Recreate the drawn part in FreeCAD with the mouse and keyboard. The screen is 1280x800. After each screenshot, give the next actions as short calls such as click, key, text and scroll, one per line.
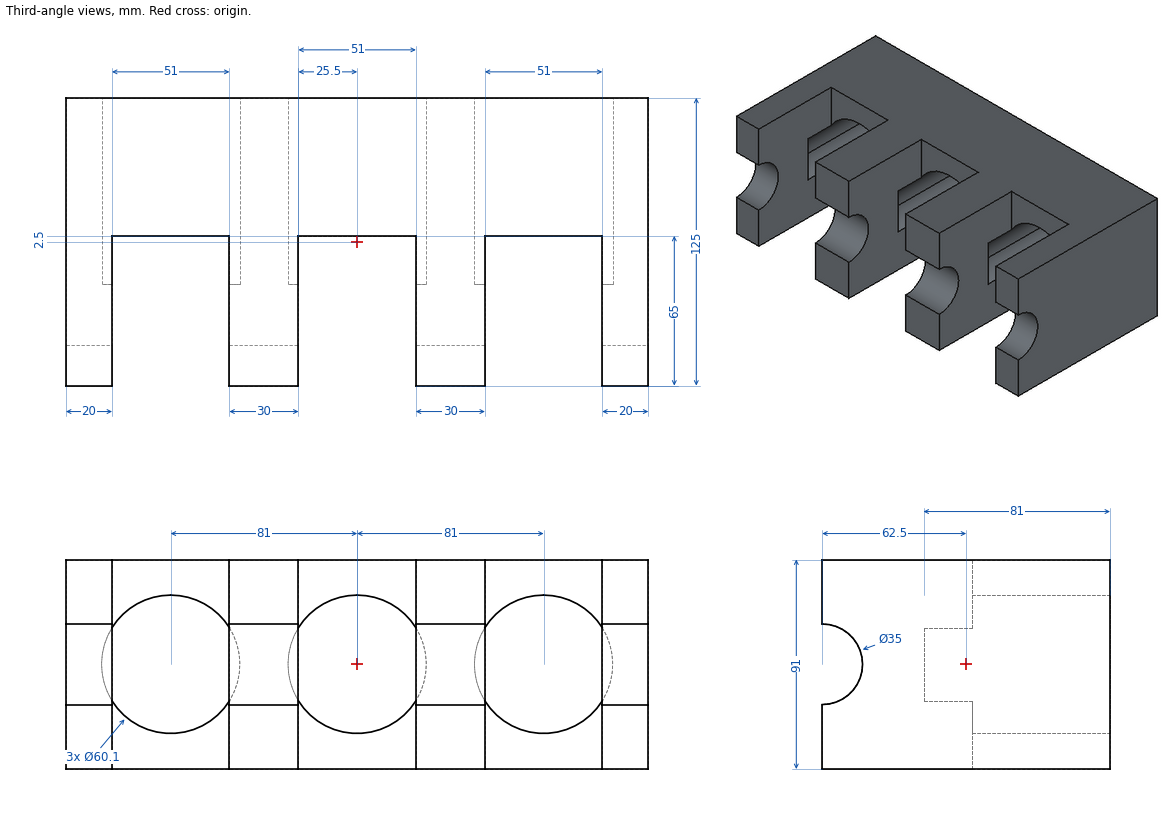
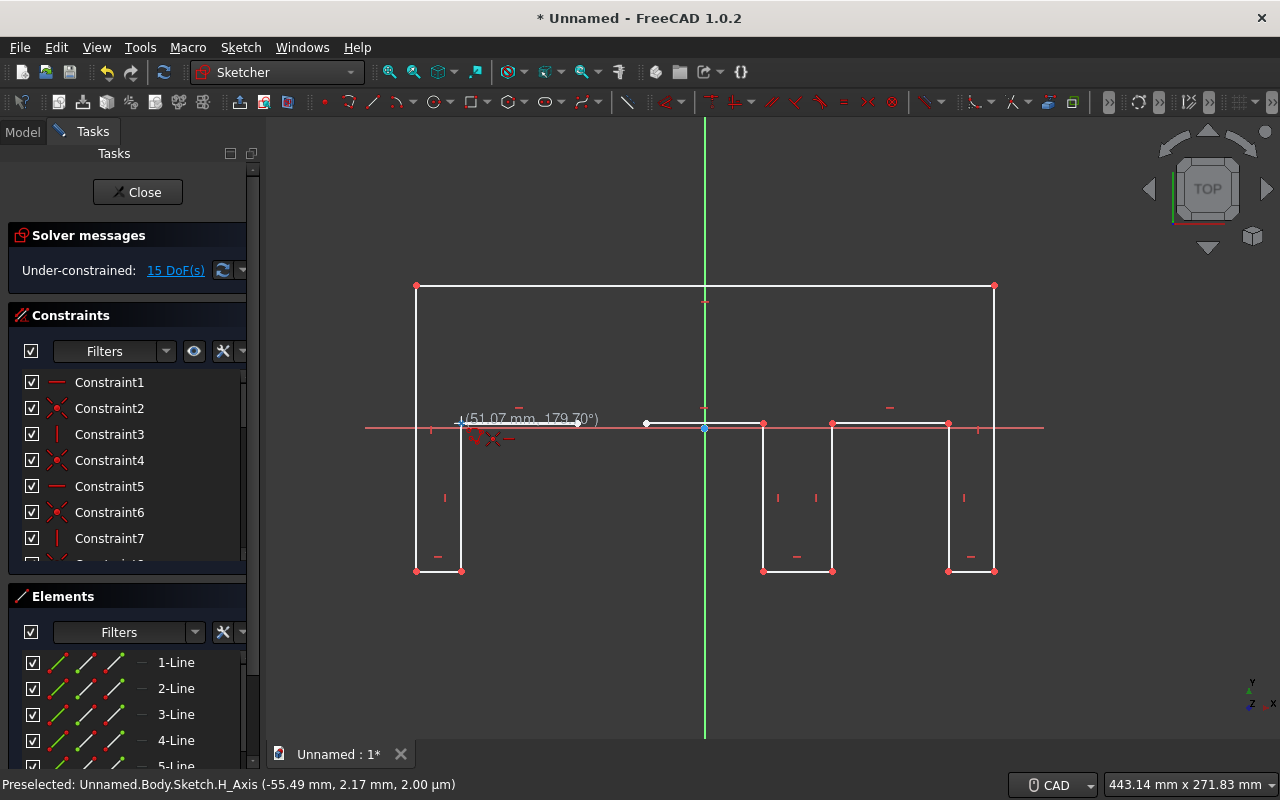
click(578, 571)
click(647, 571)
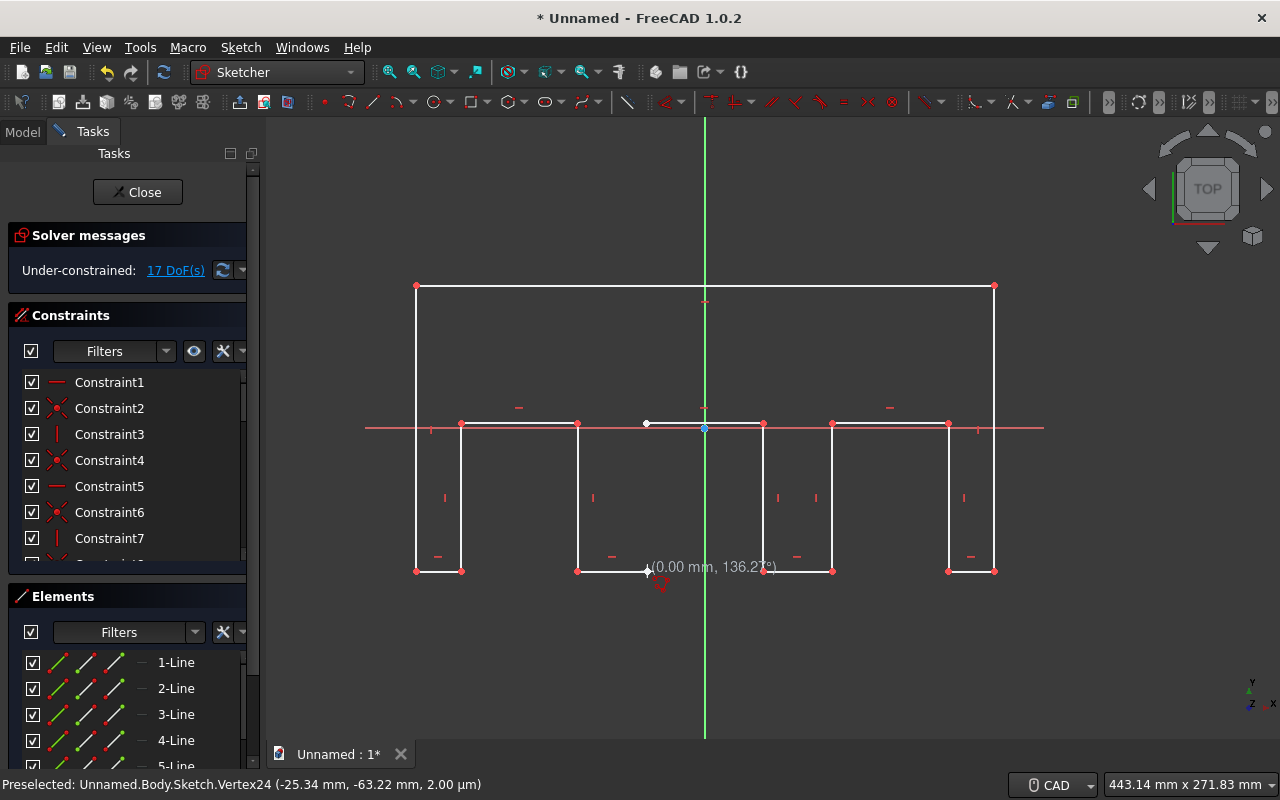
scroll(647, 423, up, 6)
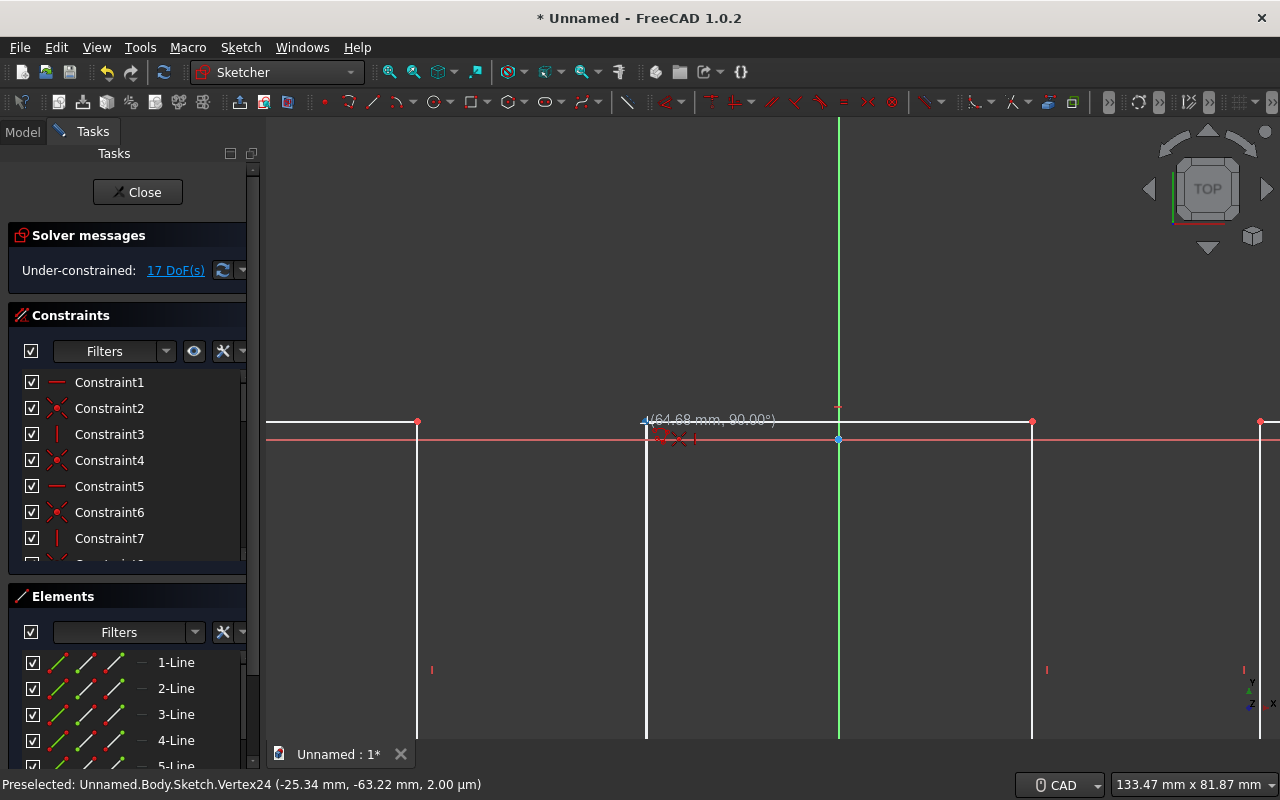
click(645, 422)
key(Escape)
key(Escape)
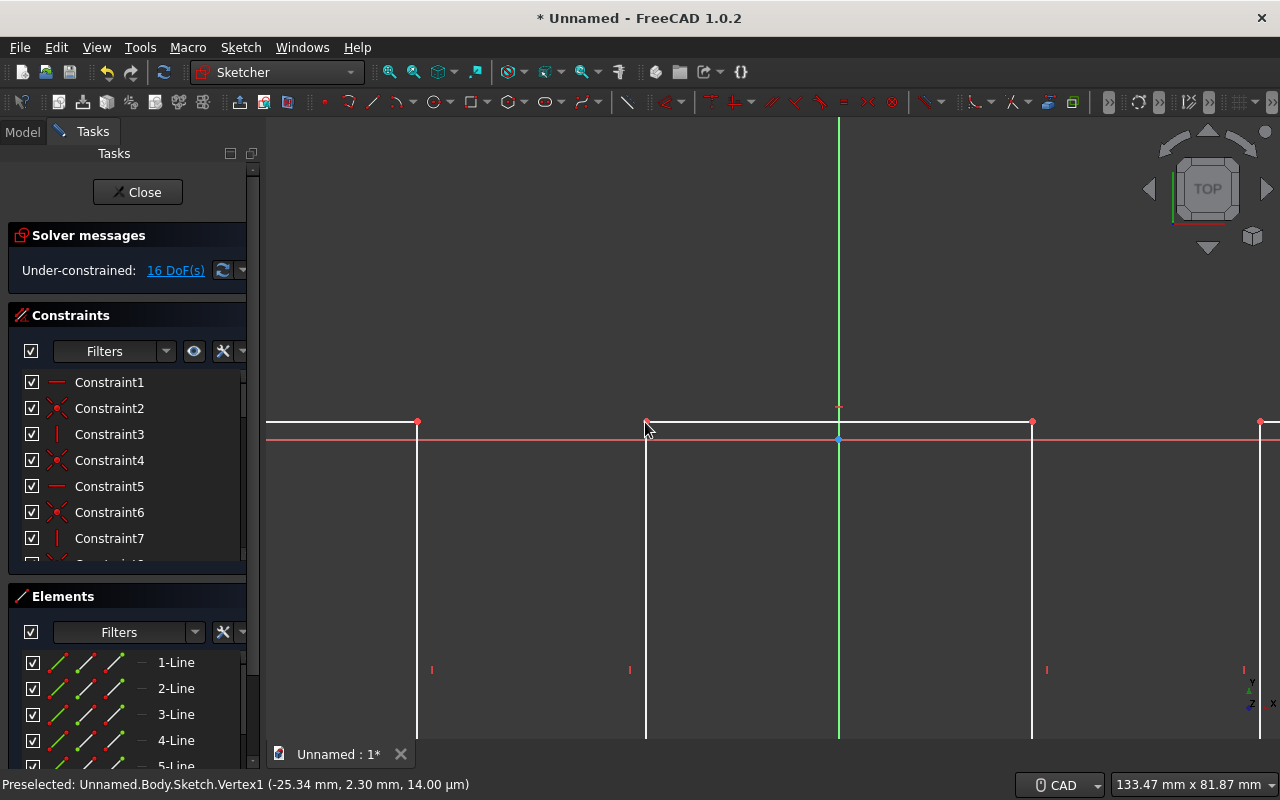
click(762, 422)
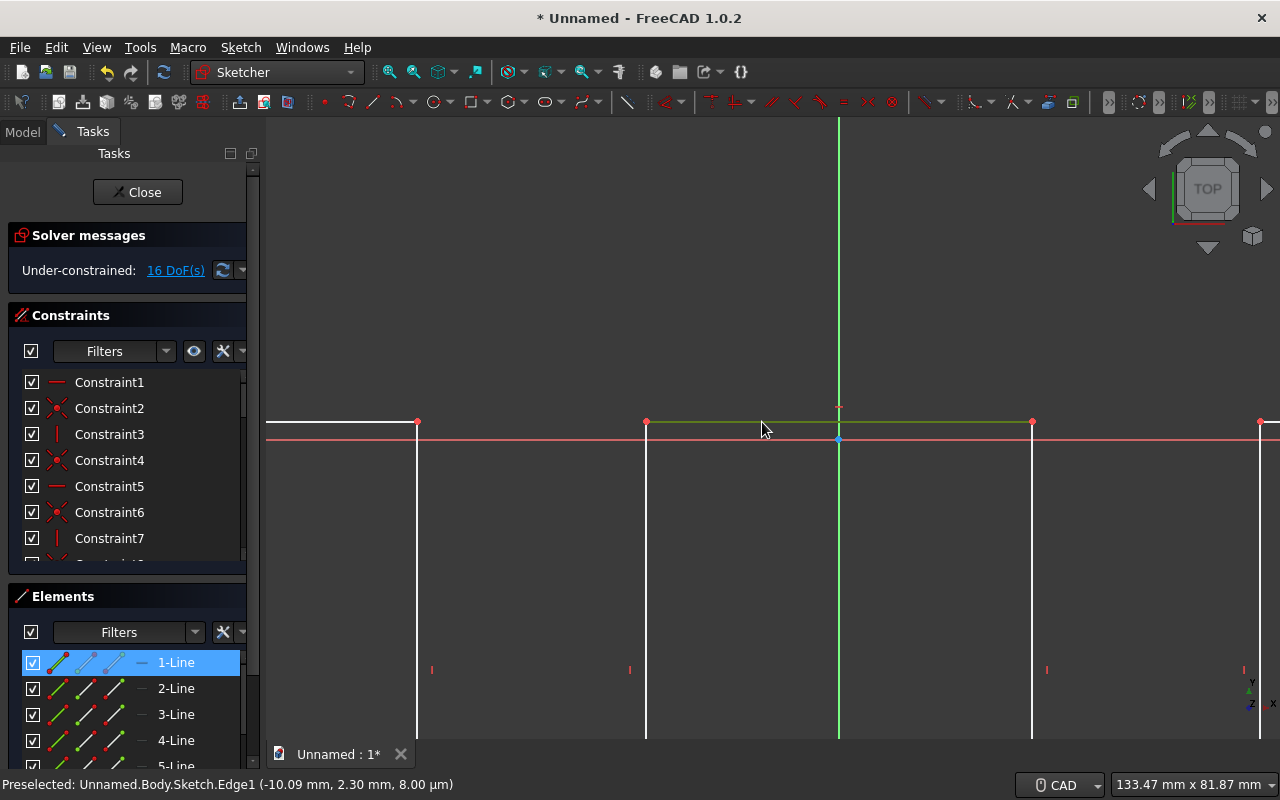
click(684, 102)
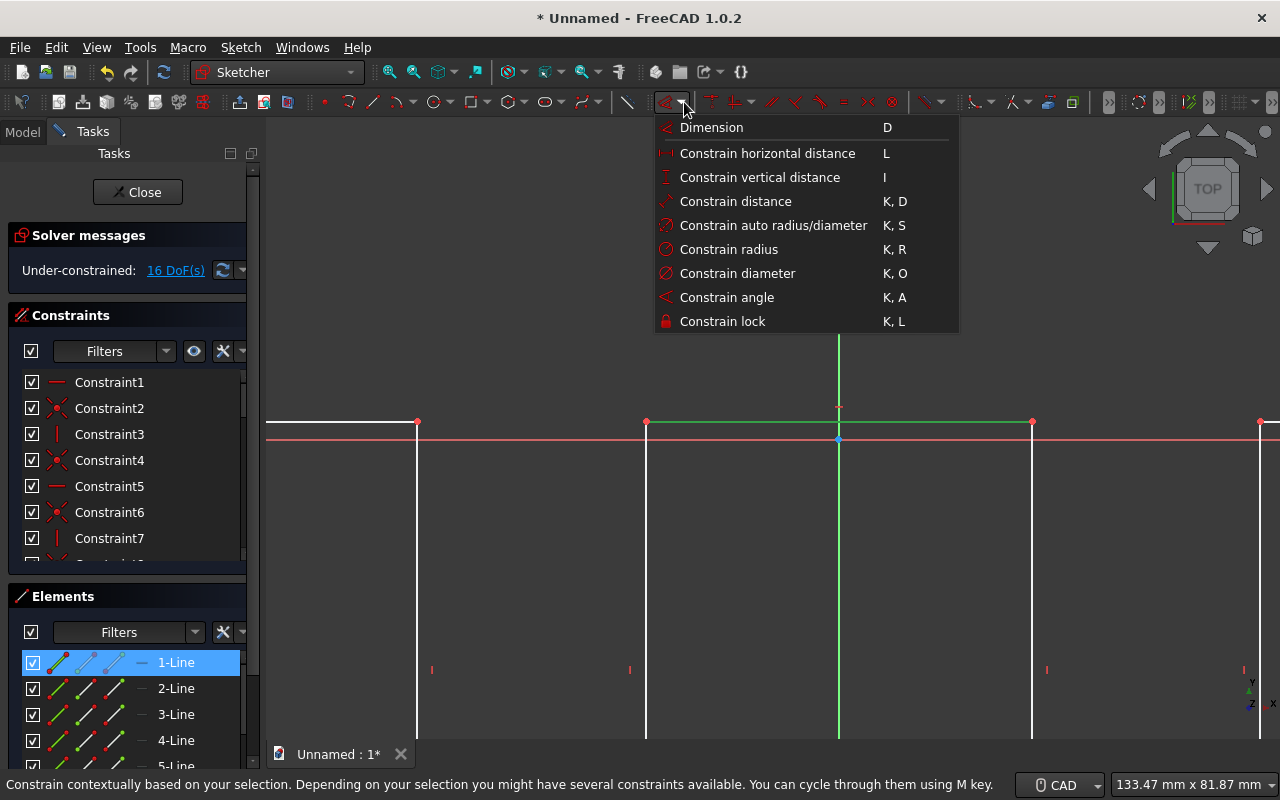
click(807, 153)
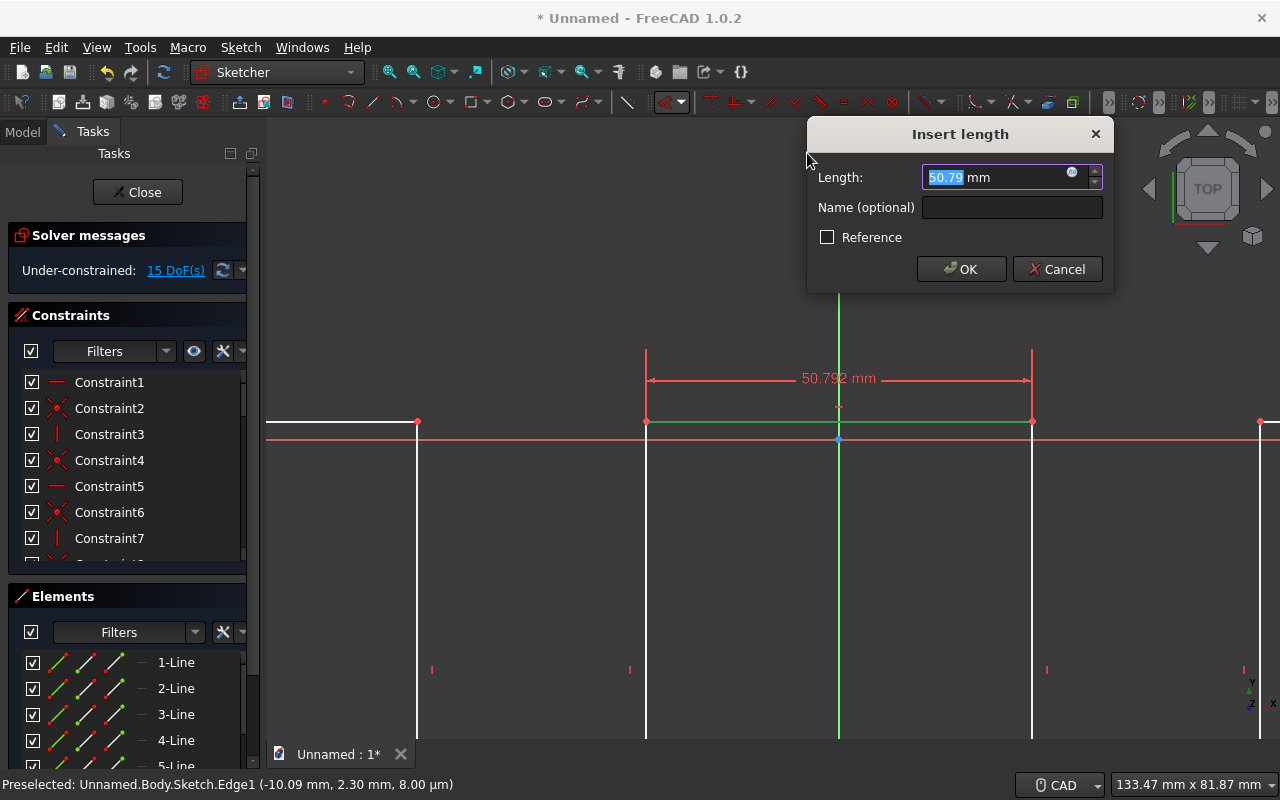
text(51)
key(Return)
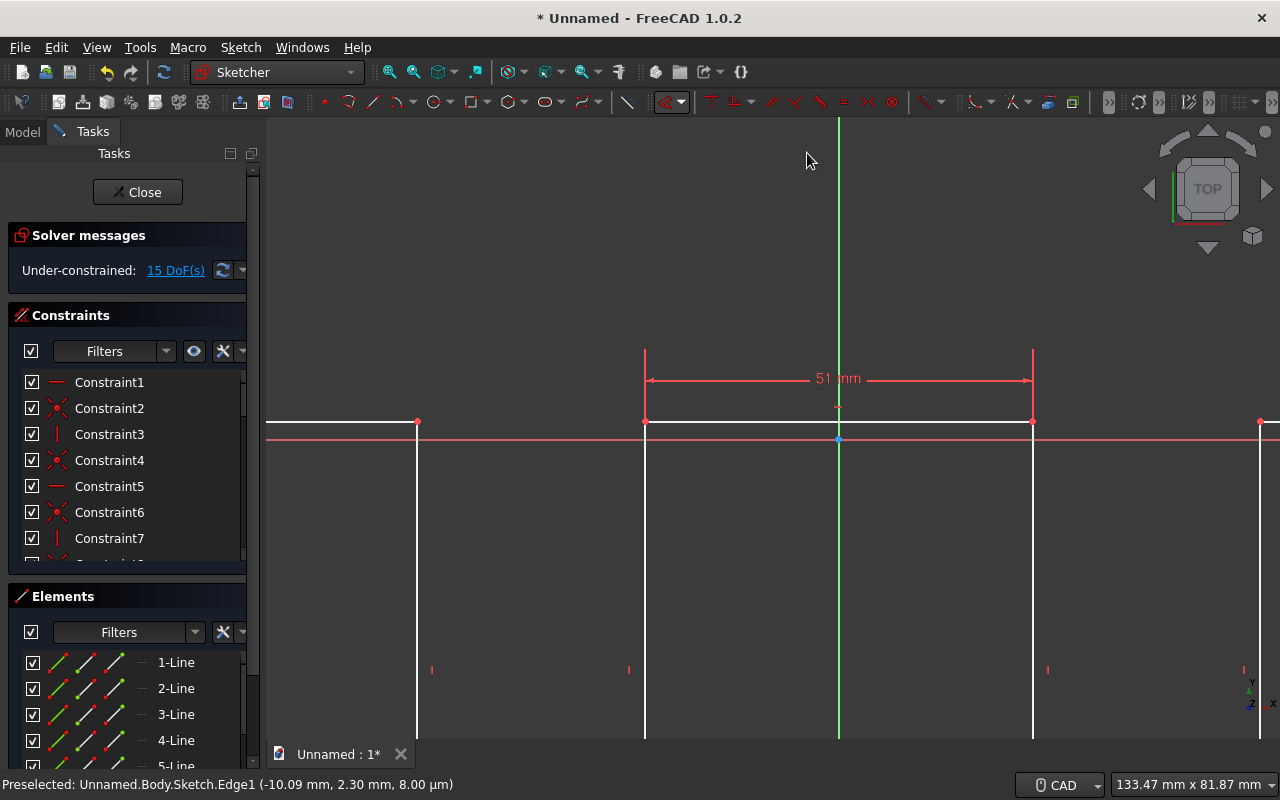
click(1033, 570)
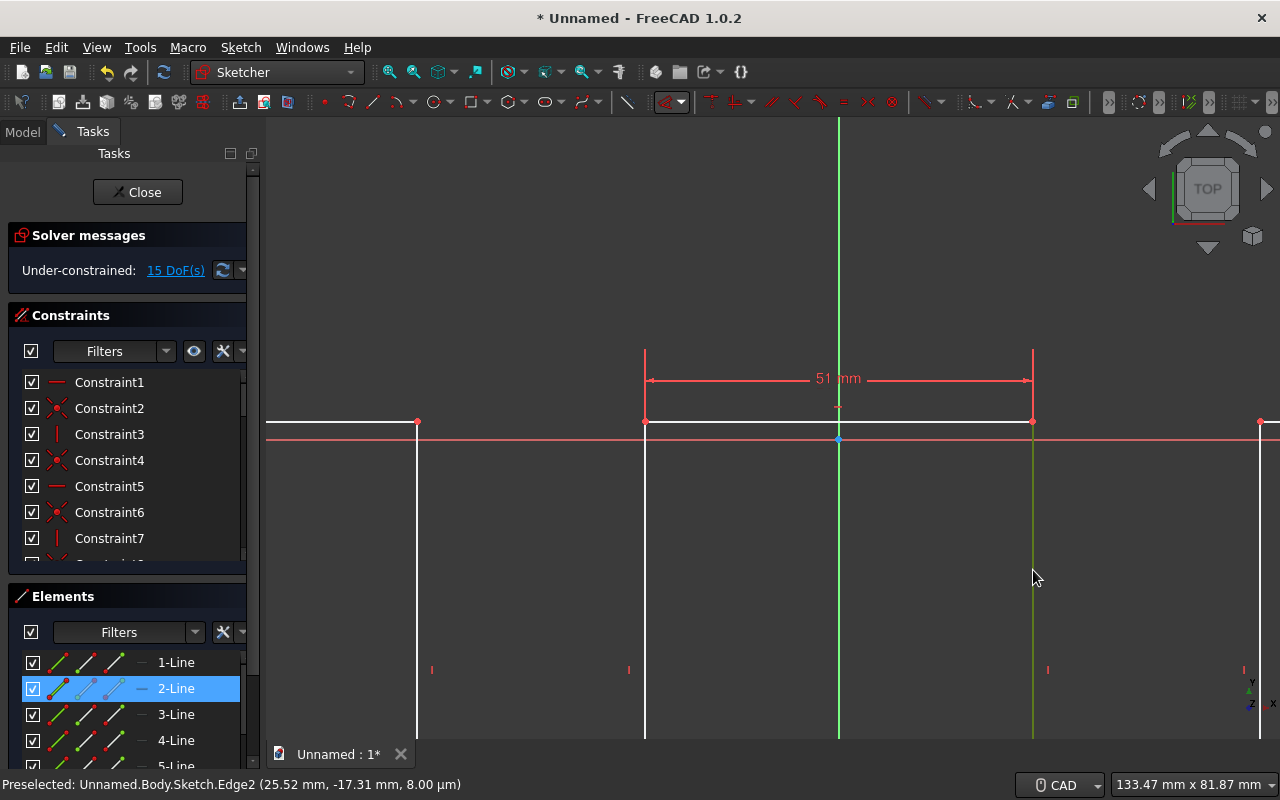
key(i)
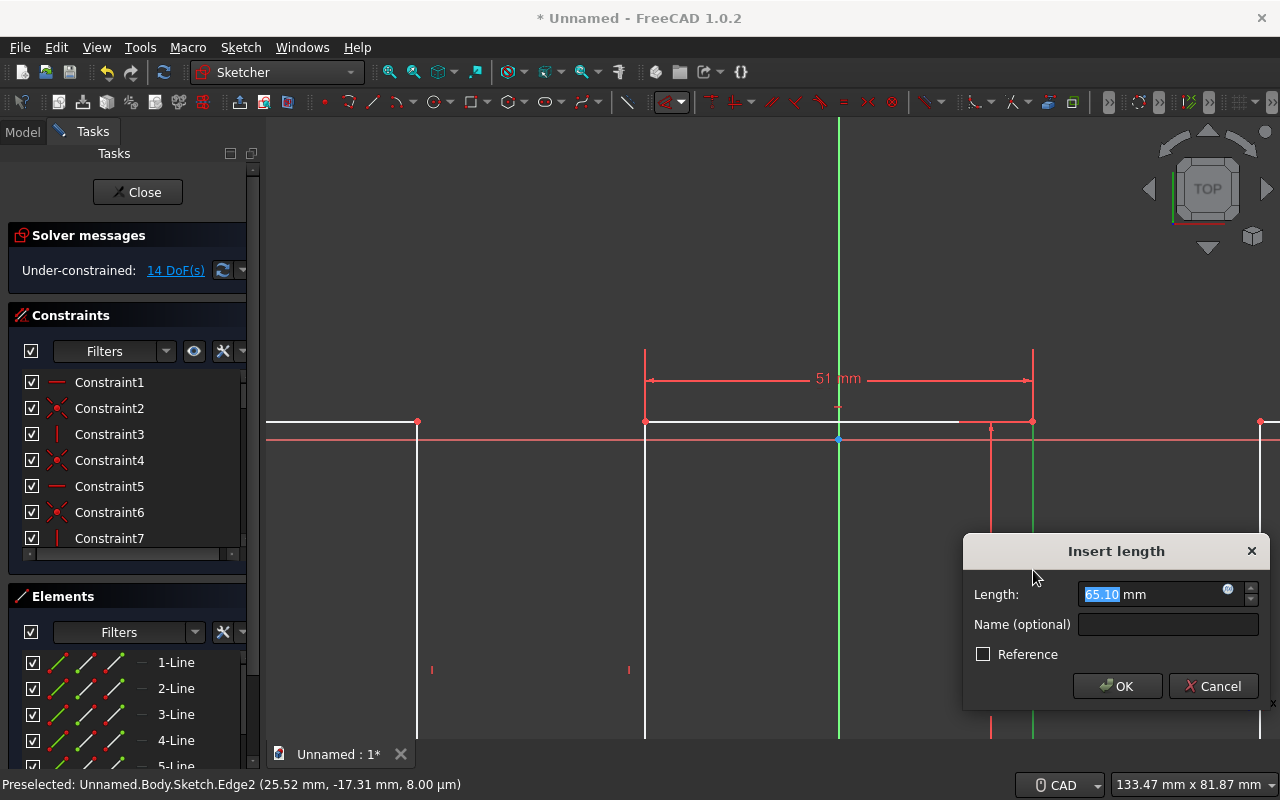
text(65)
key(Return)